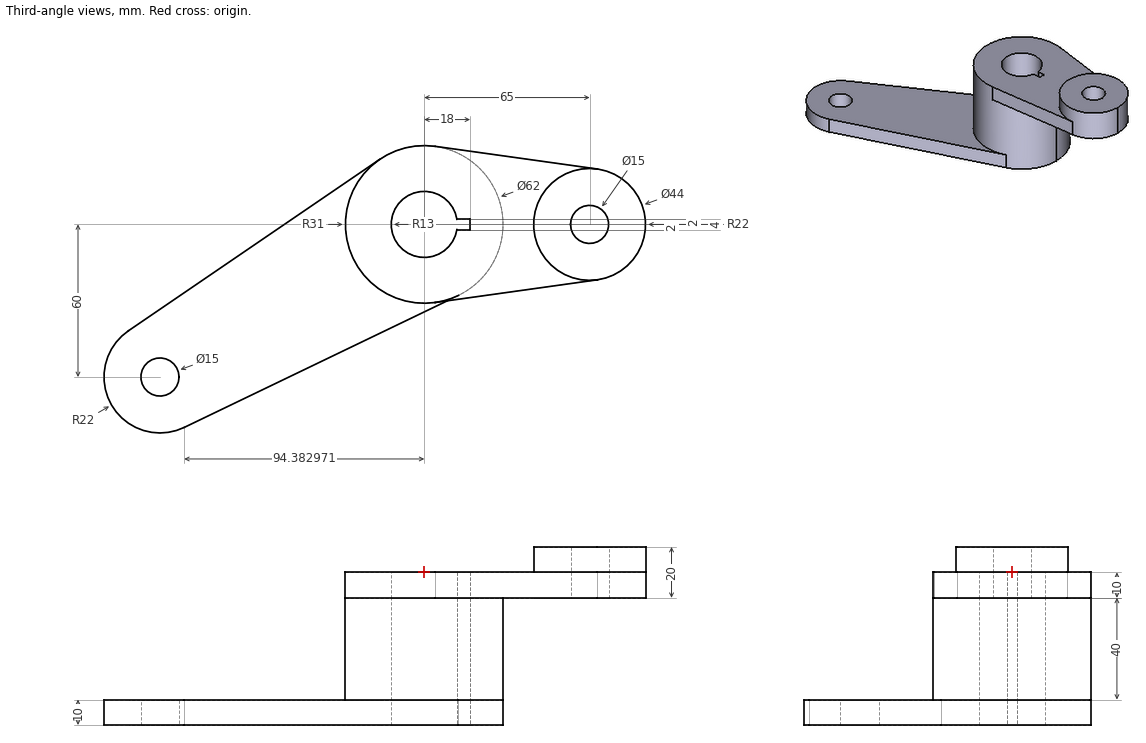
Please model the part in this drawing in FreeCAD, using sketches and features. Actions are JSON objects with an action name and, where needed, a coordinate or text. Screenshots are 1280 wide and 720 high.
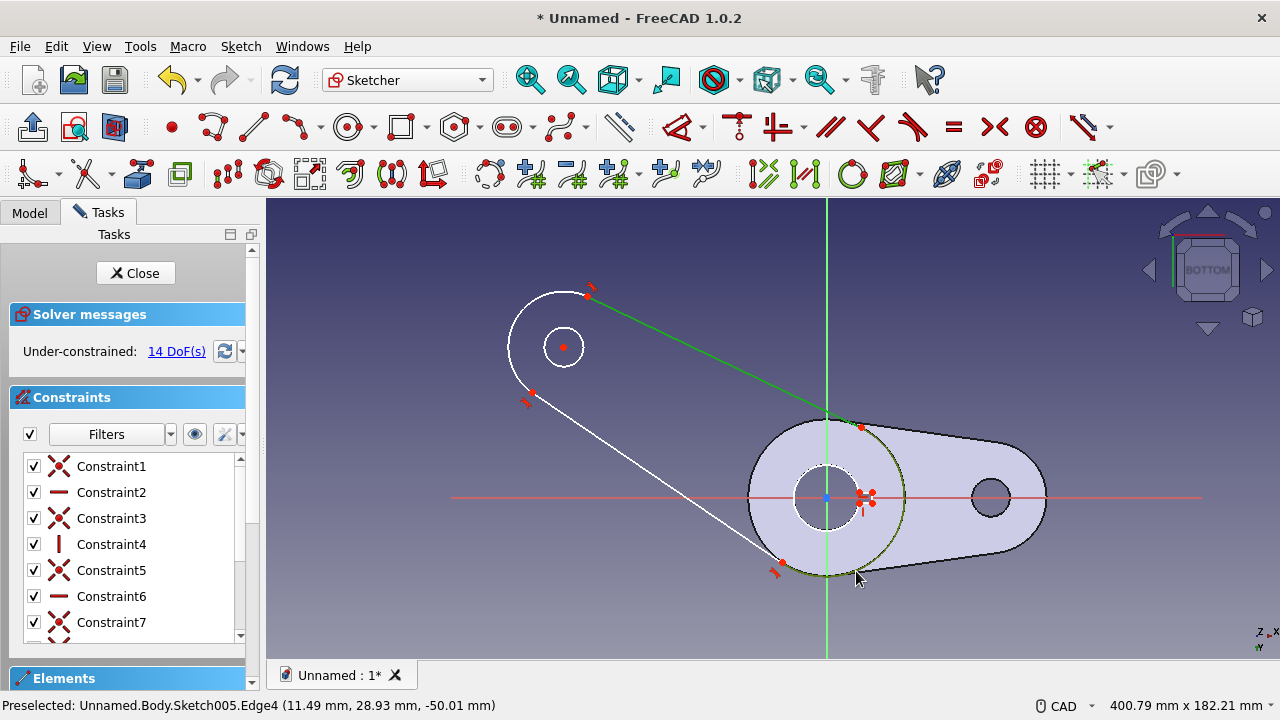
{"action": "left_click", "coordinate": [913, 128]}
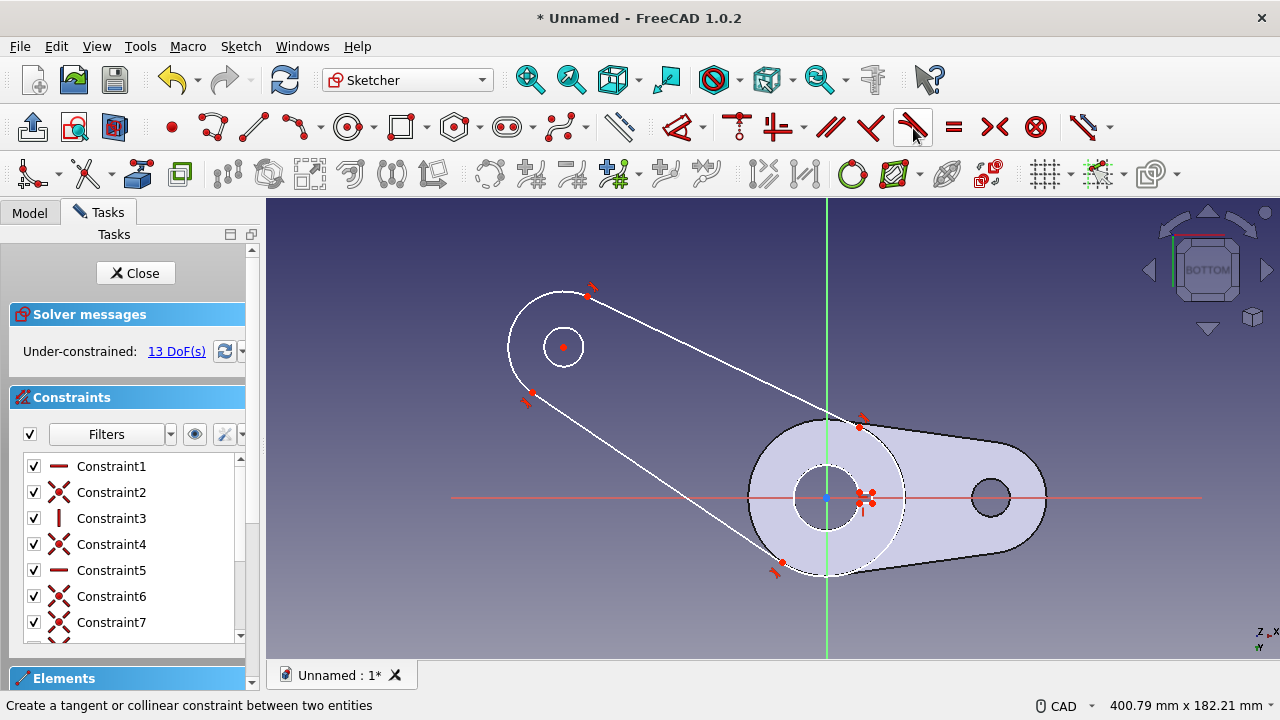
{"action": "left_click", "coordinate": [856, 571]}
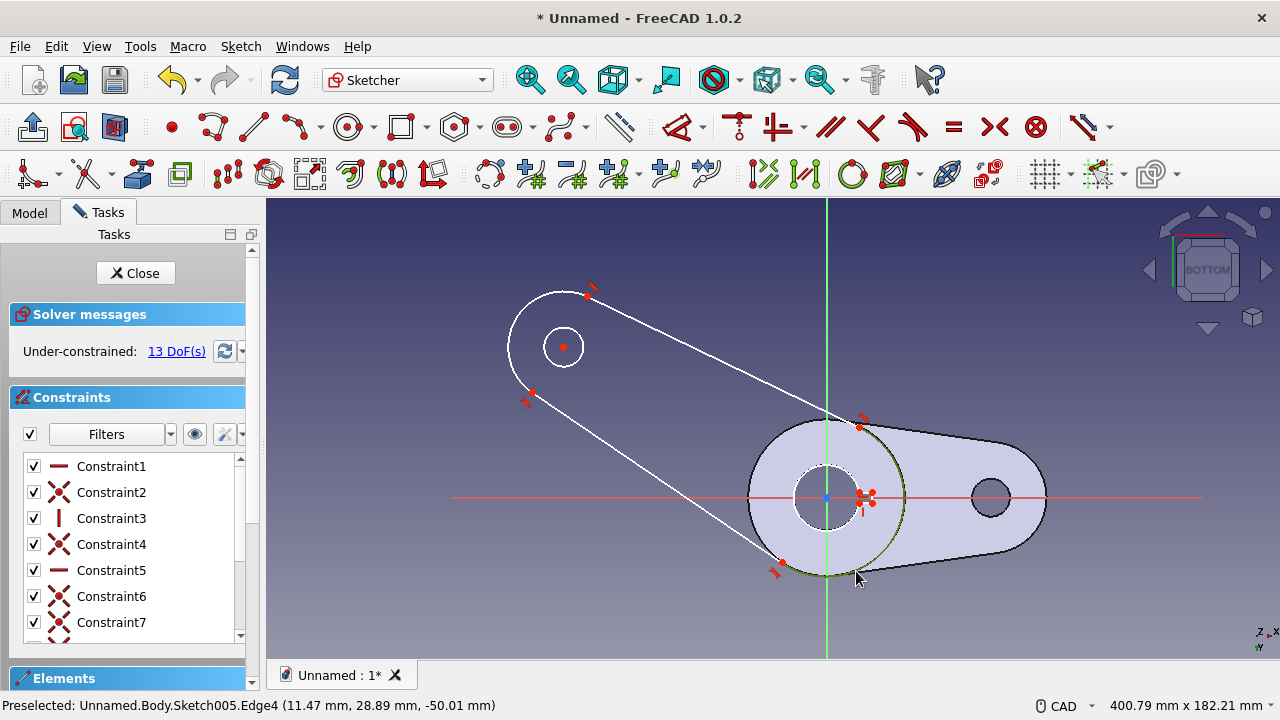
{"action": "left_click", "coordinate": [814, 467]}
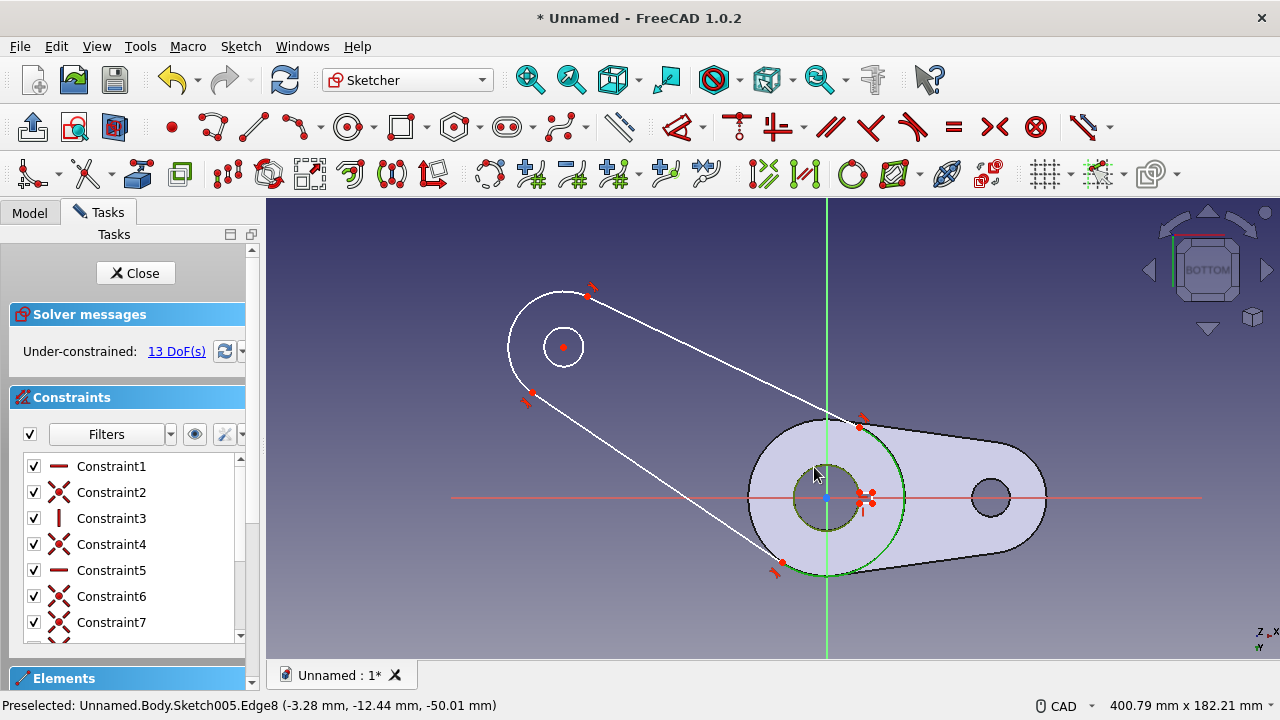
{"action": "key", "text": "c"}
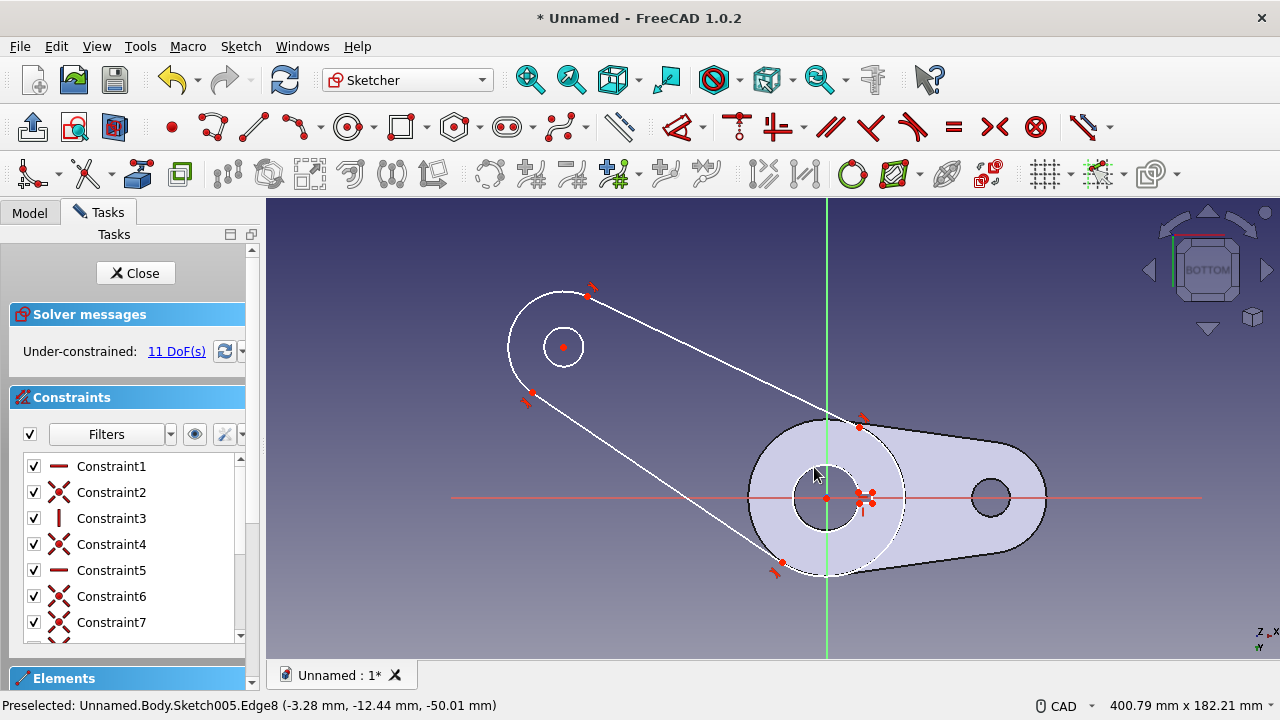
{"action": "scroll", "coordinate": [826, 498], "scroll_direction": "up", "scroll_amount": 4}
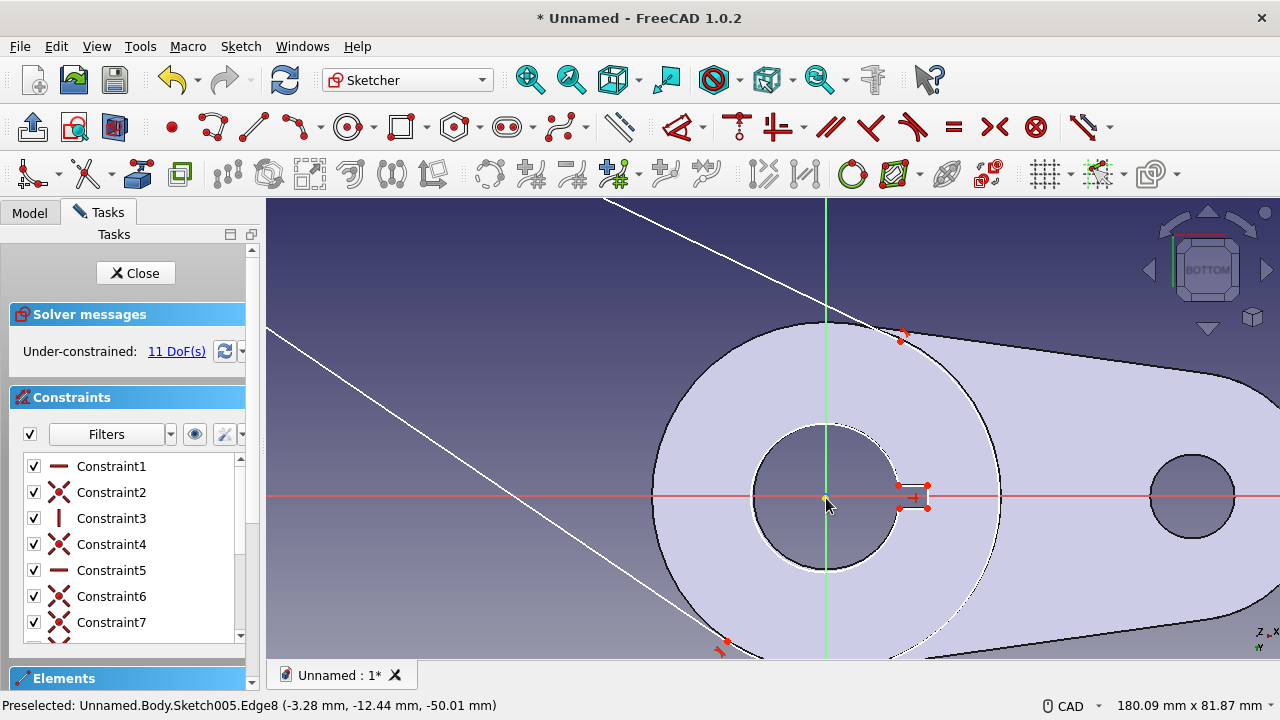
{"action": "left_click_drag", "start_coordinate": [815, 486], "coordinate": [836, 508]}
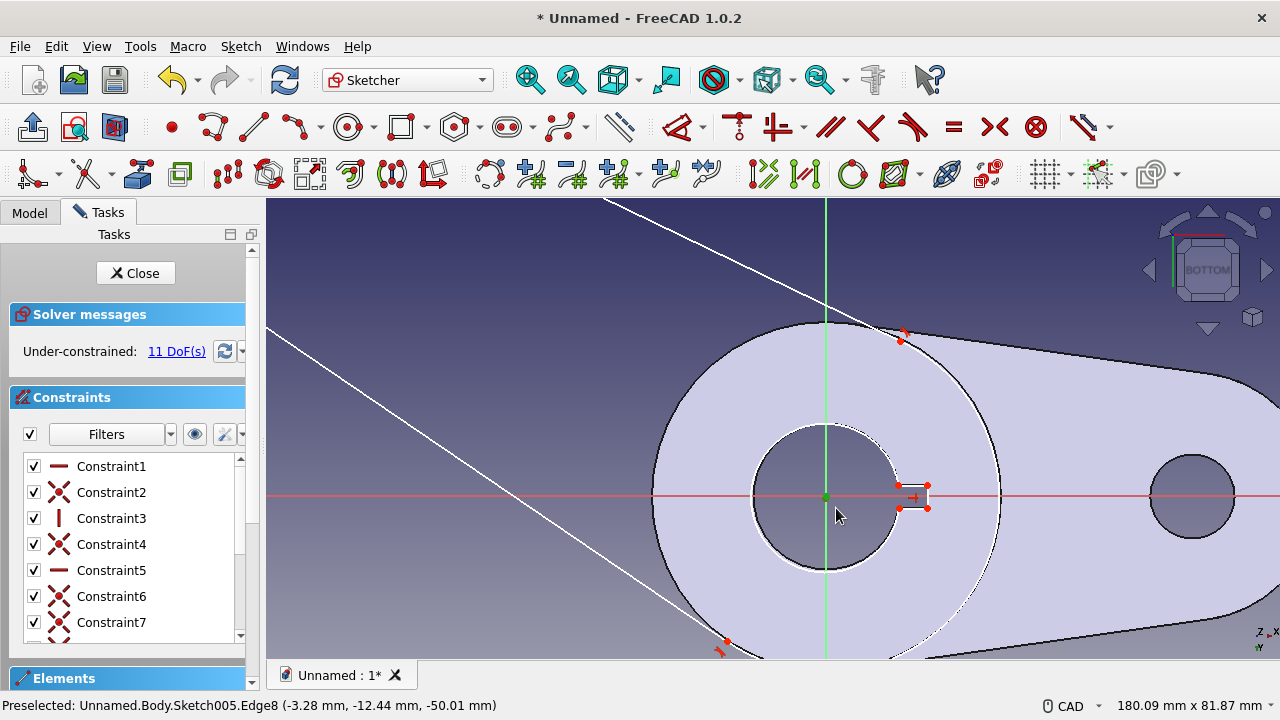
{"action": "left_click", "coordinate": [737, 128]}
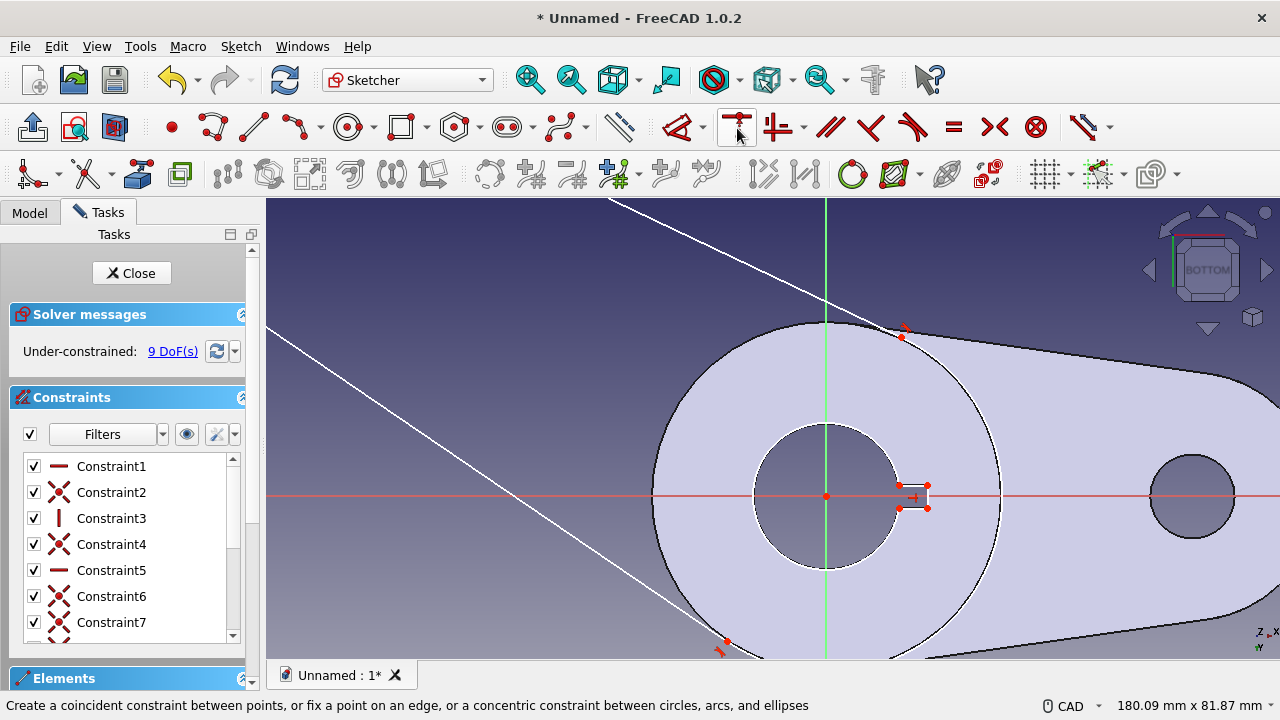
{"action": "key", "text": "d"}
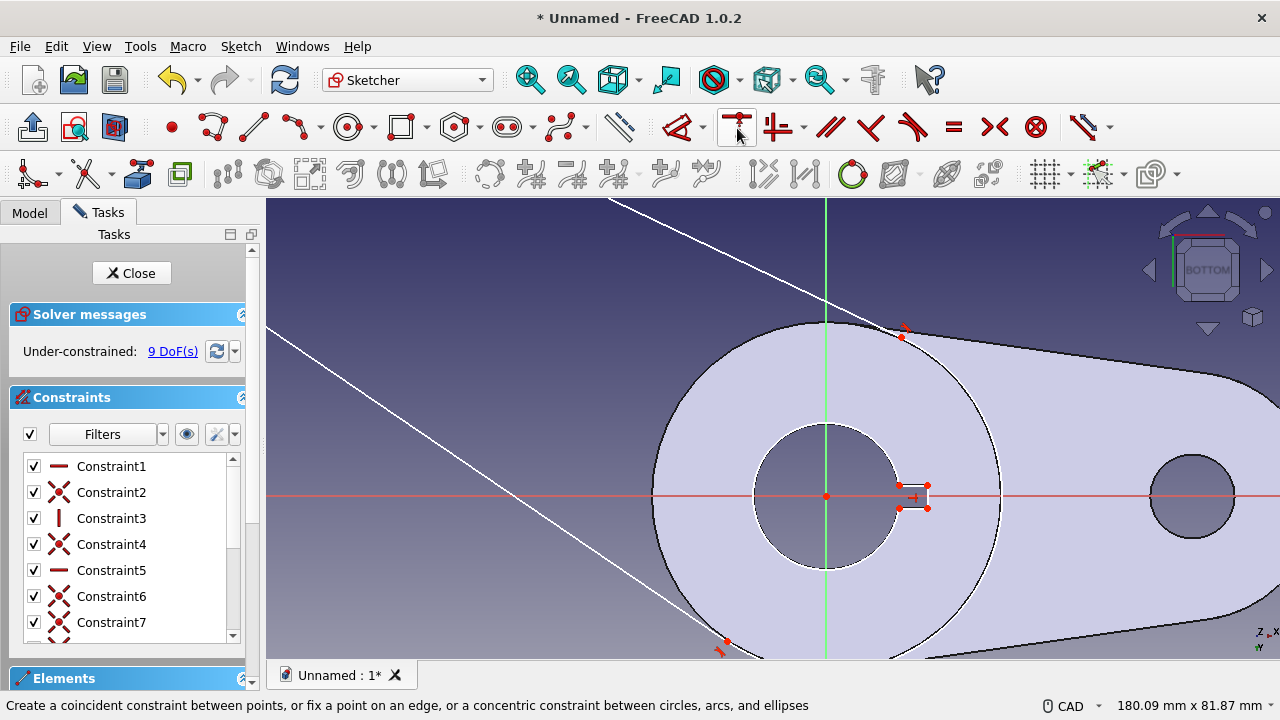
{"action": "scroll", "coordinate": [826, 498], "scroll_direction": "down", "scroll_amount": 4}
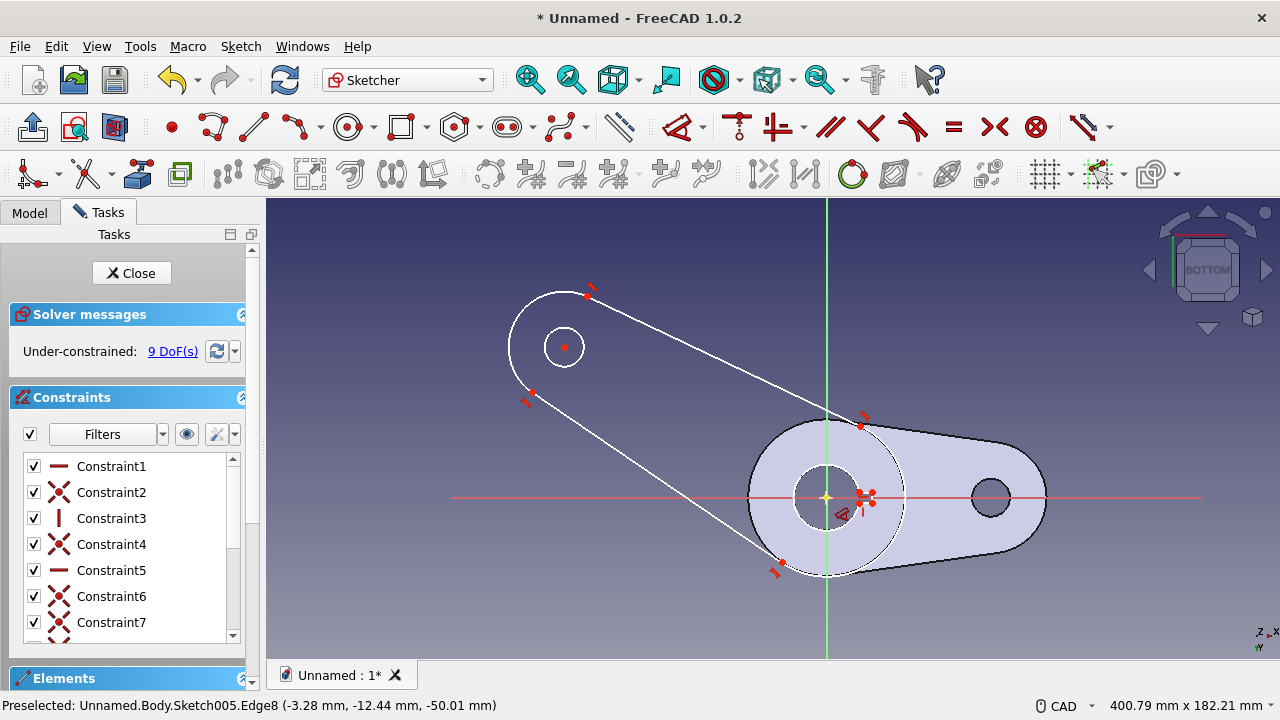
{"action": "left_click", "coordinate": [540, 297]}
{"action": "left_click", "coordinate": [526, 268]}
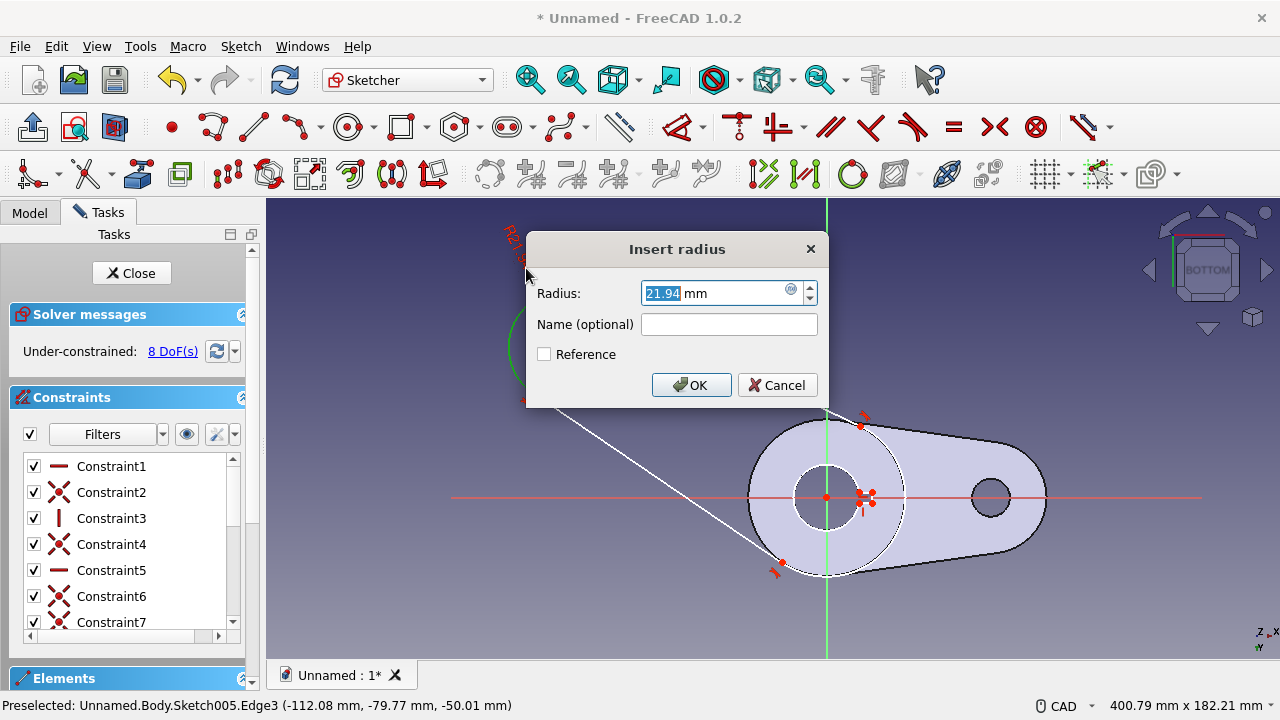
{"action": "type", "text": "22"}
{"action": "key", "text": "Return"}